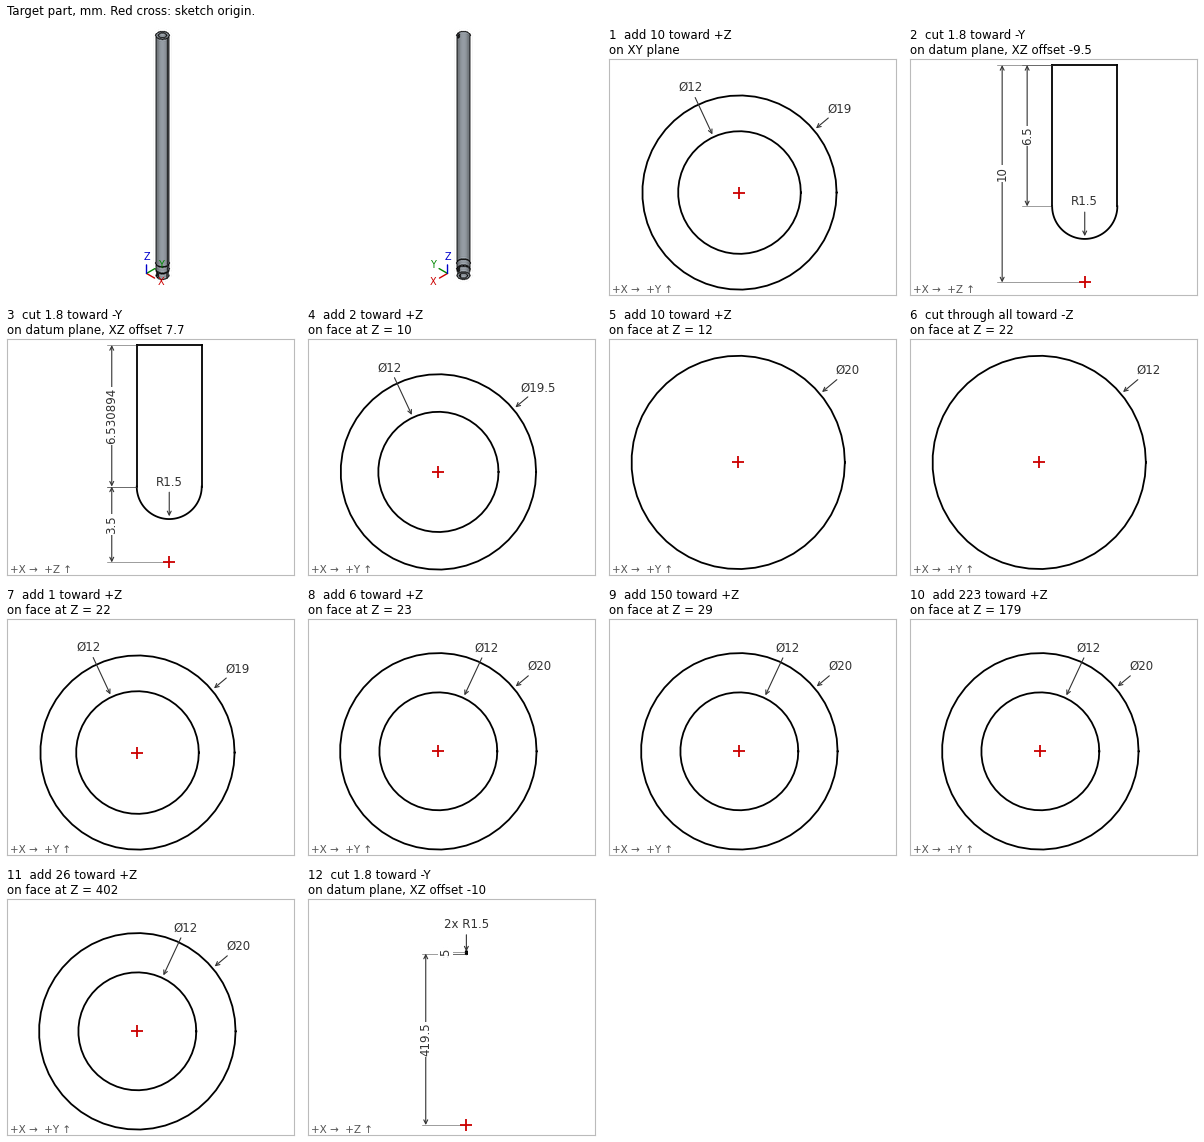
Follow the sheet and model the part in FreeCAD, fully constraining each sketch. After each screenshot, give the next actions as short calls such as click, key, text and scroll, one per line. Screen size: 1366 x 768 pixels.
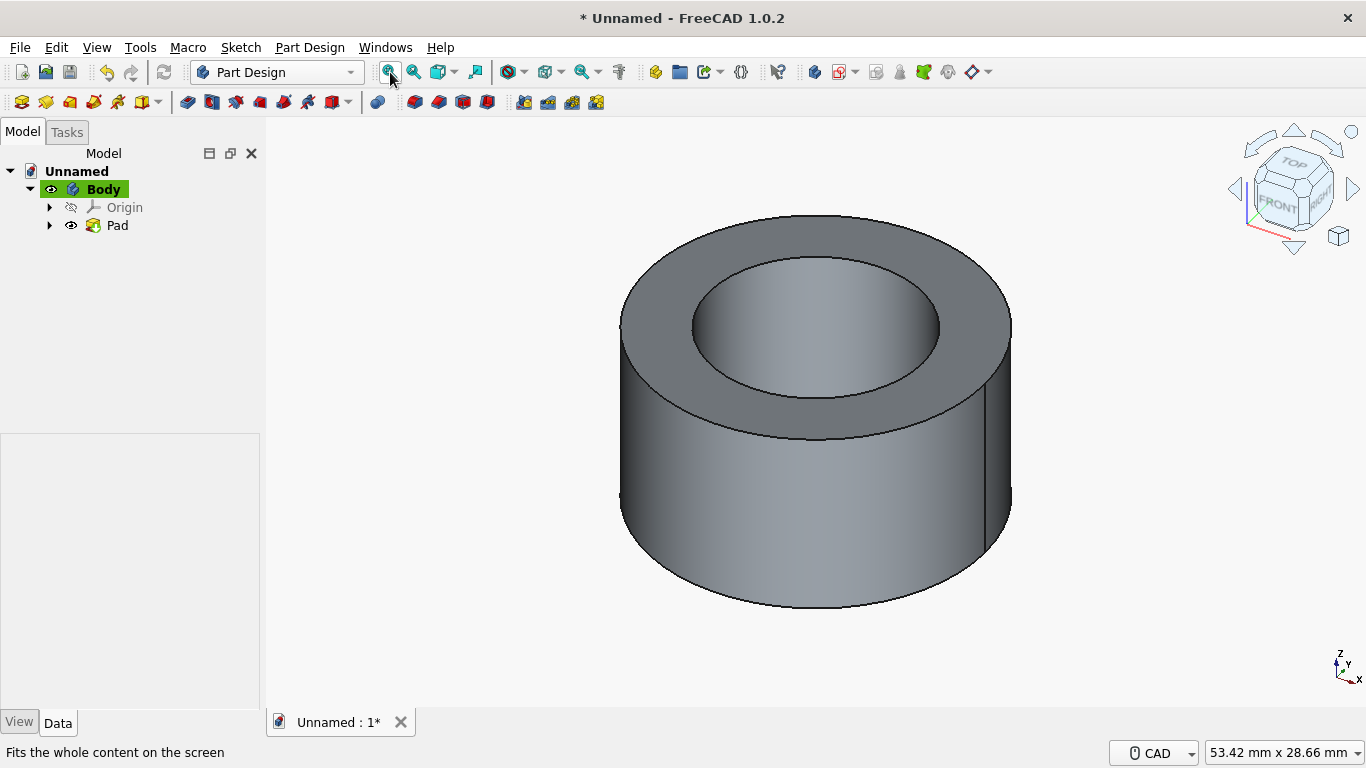
click(50, 207)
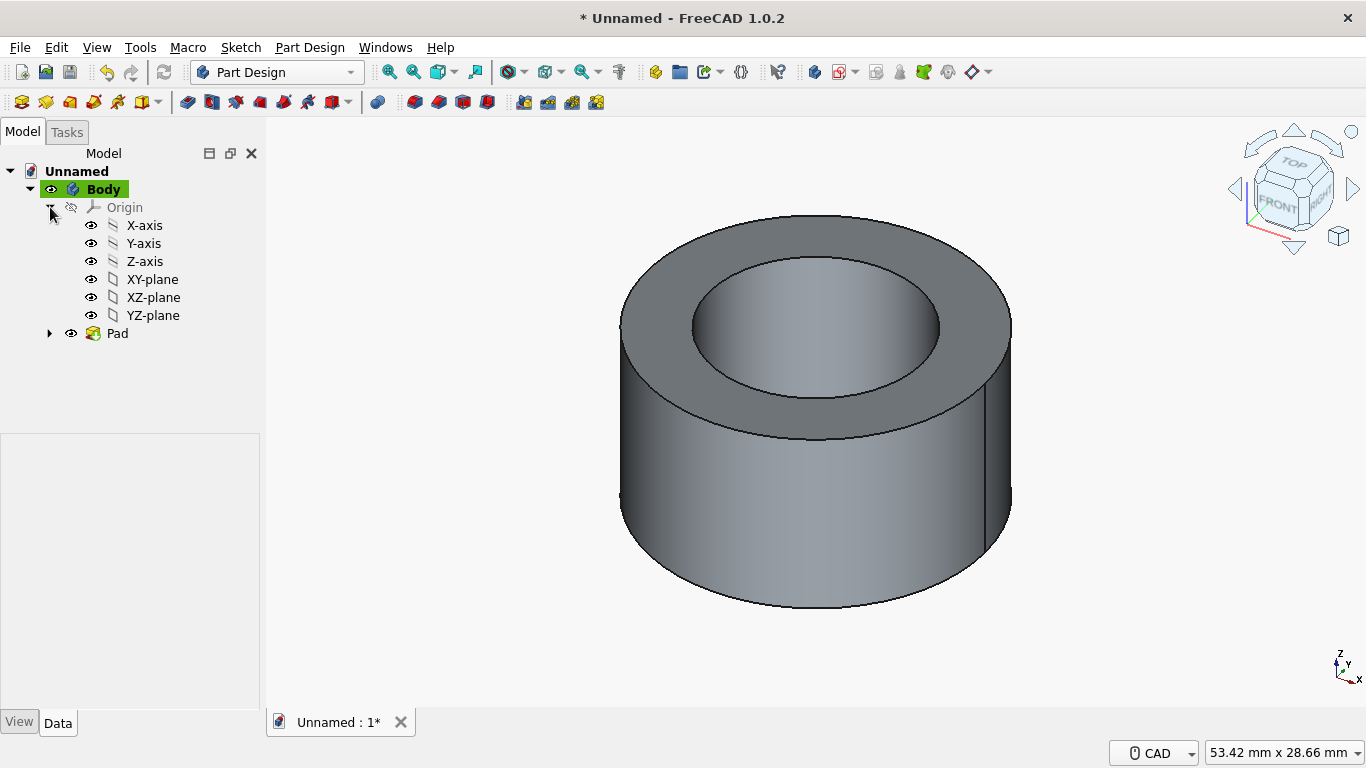
click(136, 297)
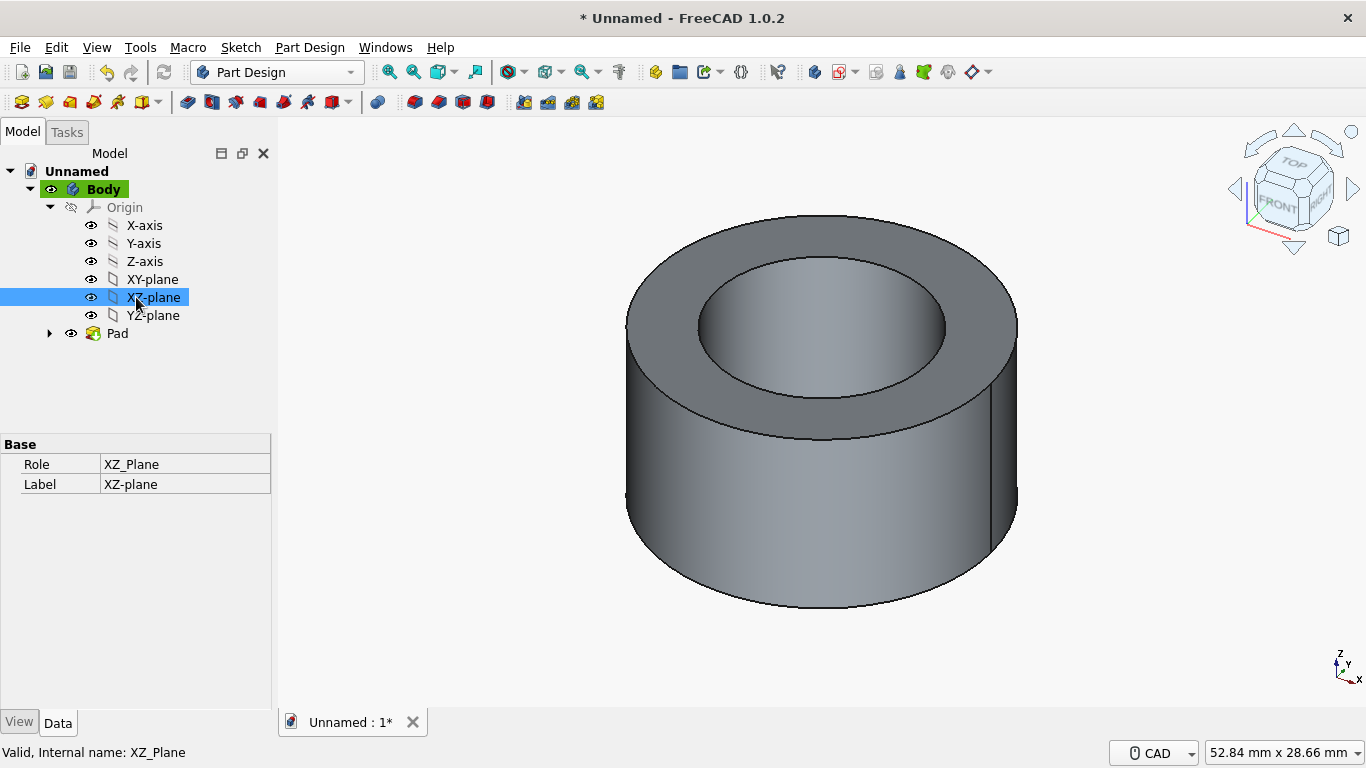
click(972, 72)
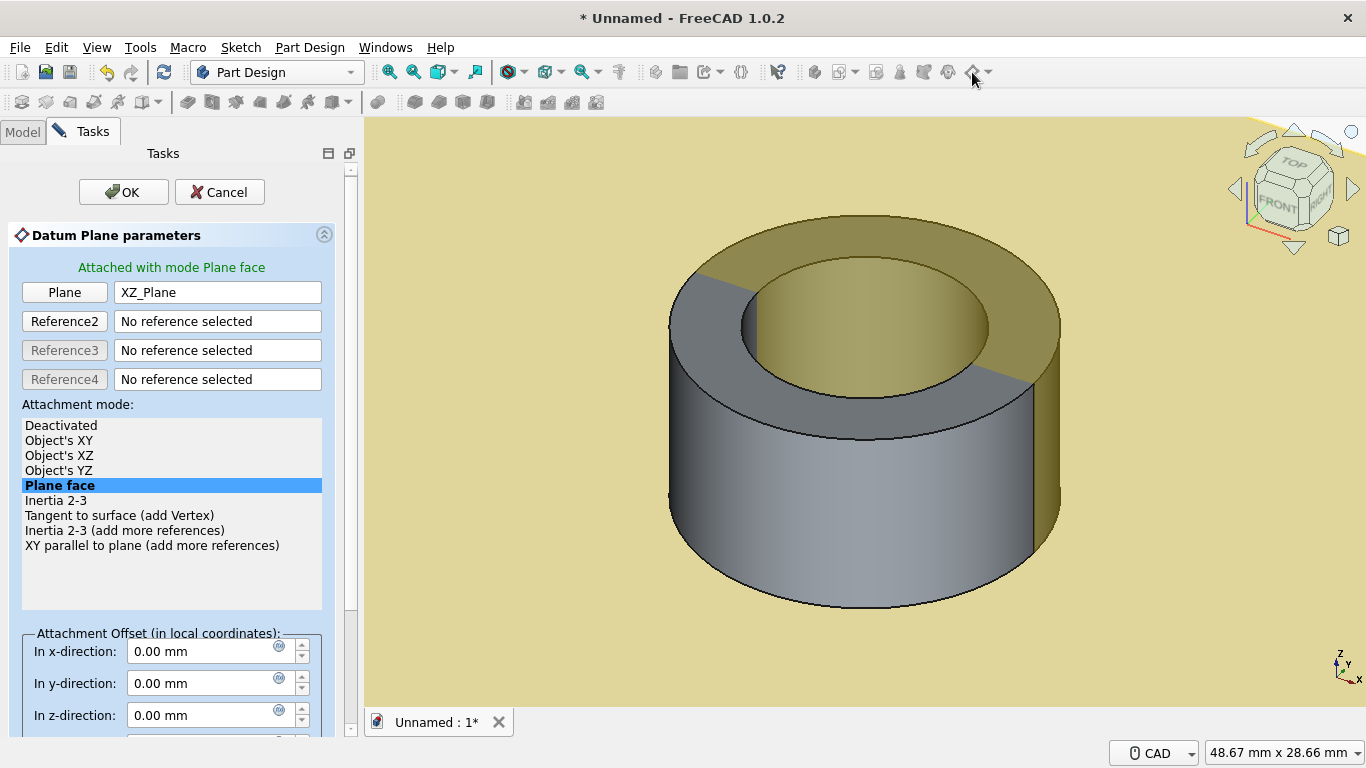
triple_click(210, 715)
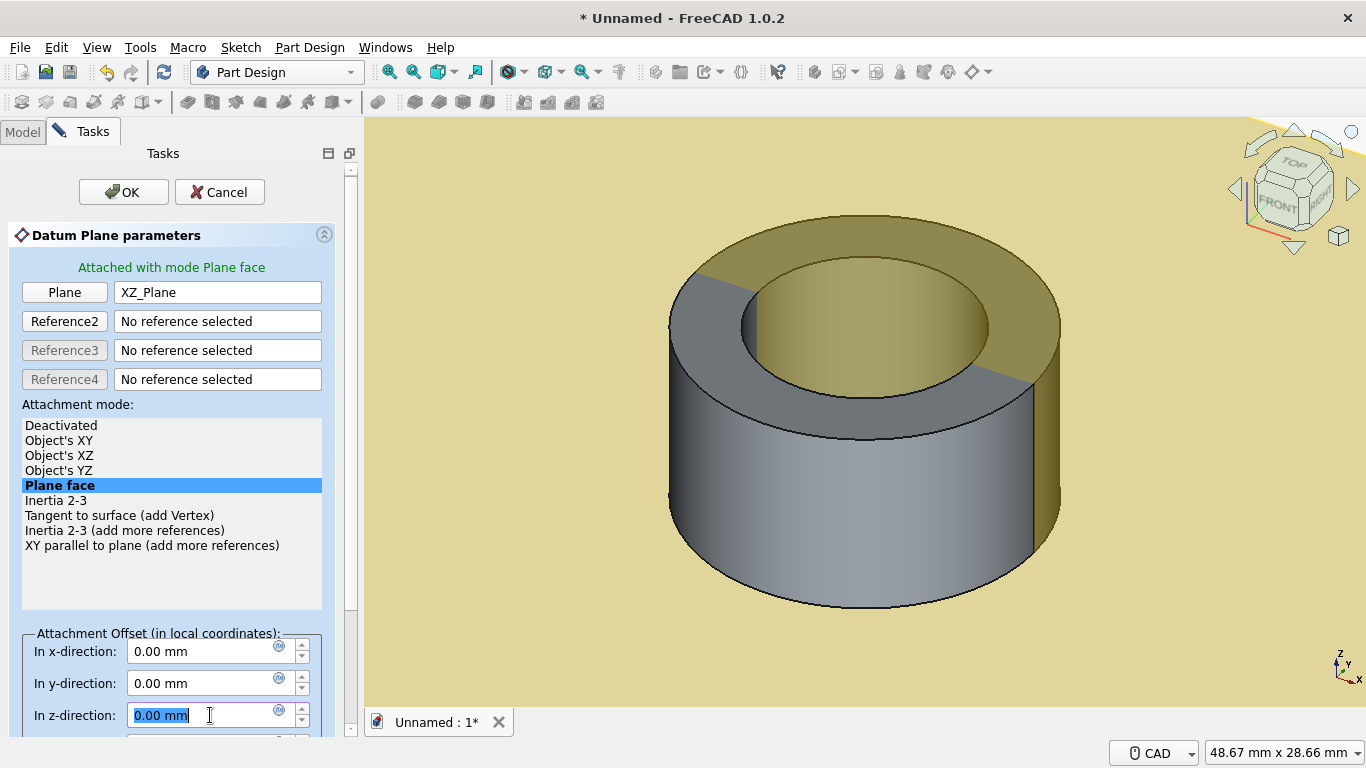
text(-9.5)
key(Tab)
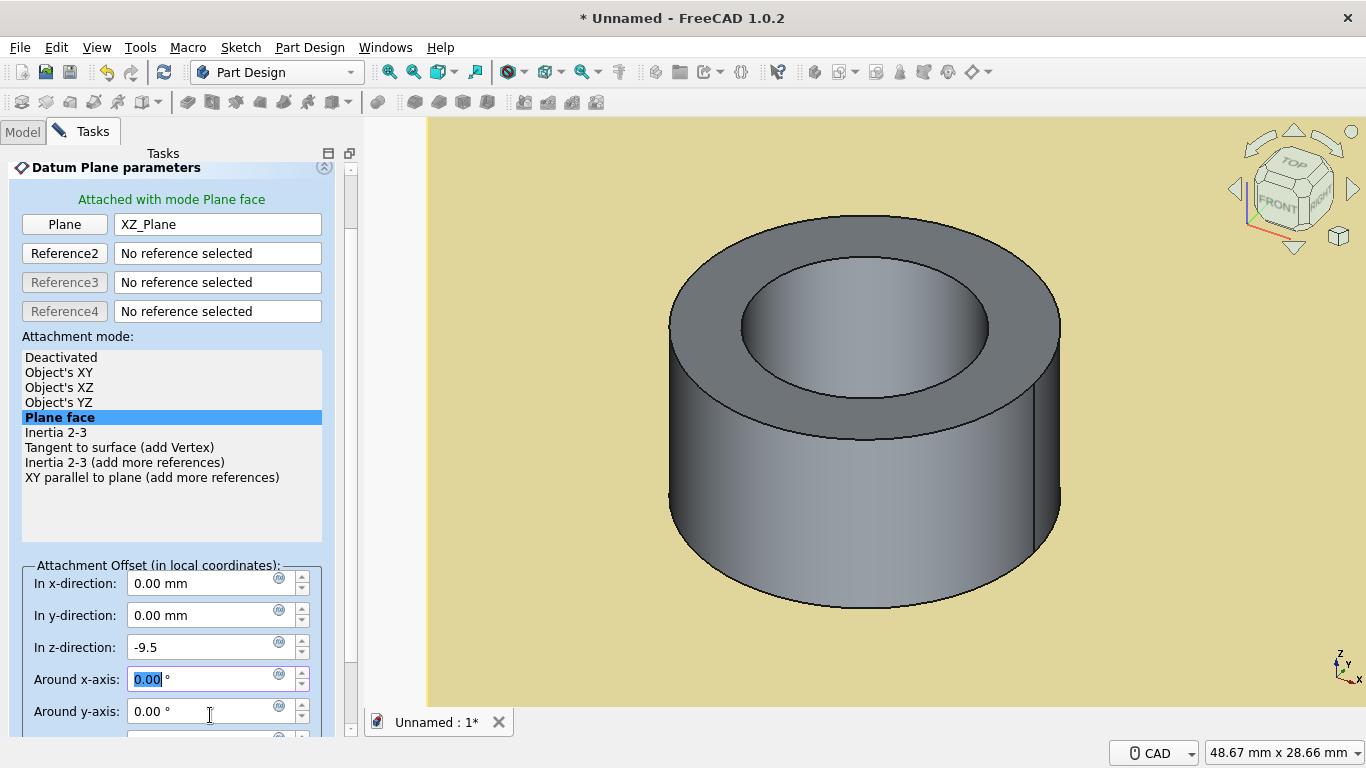
scroll(351, 450, up, 2)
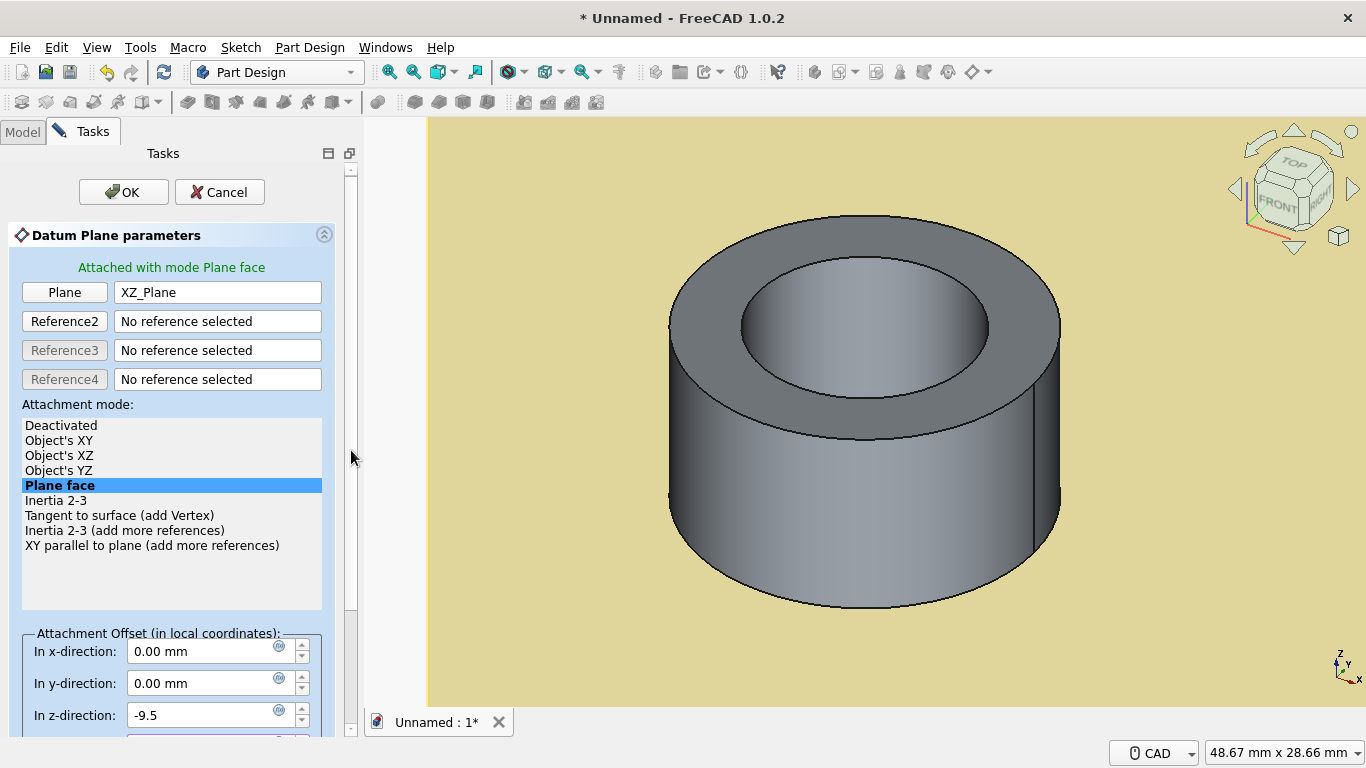
click(124, 192)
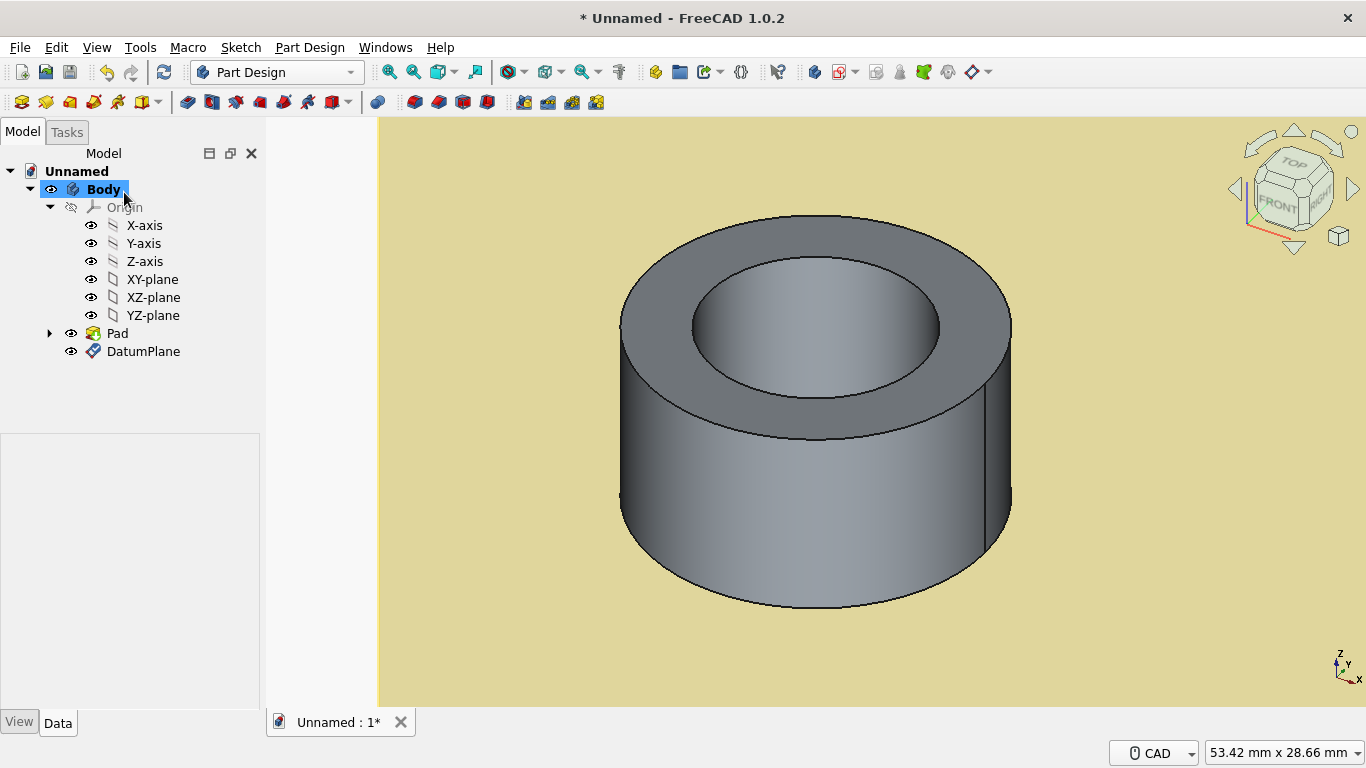
click(116, 351)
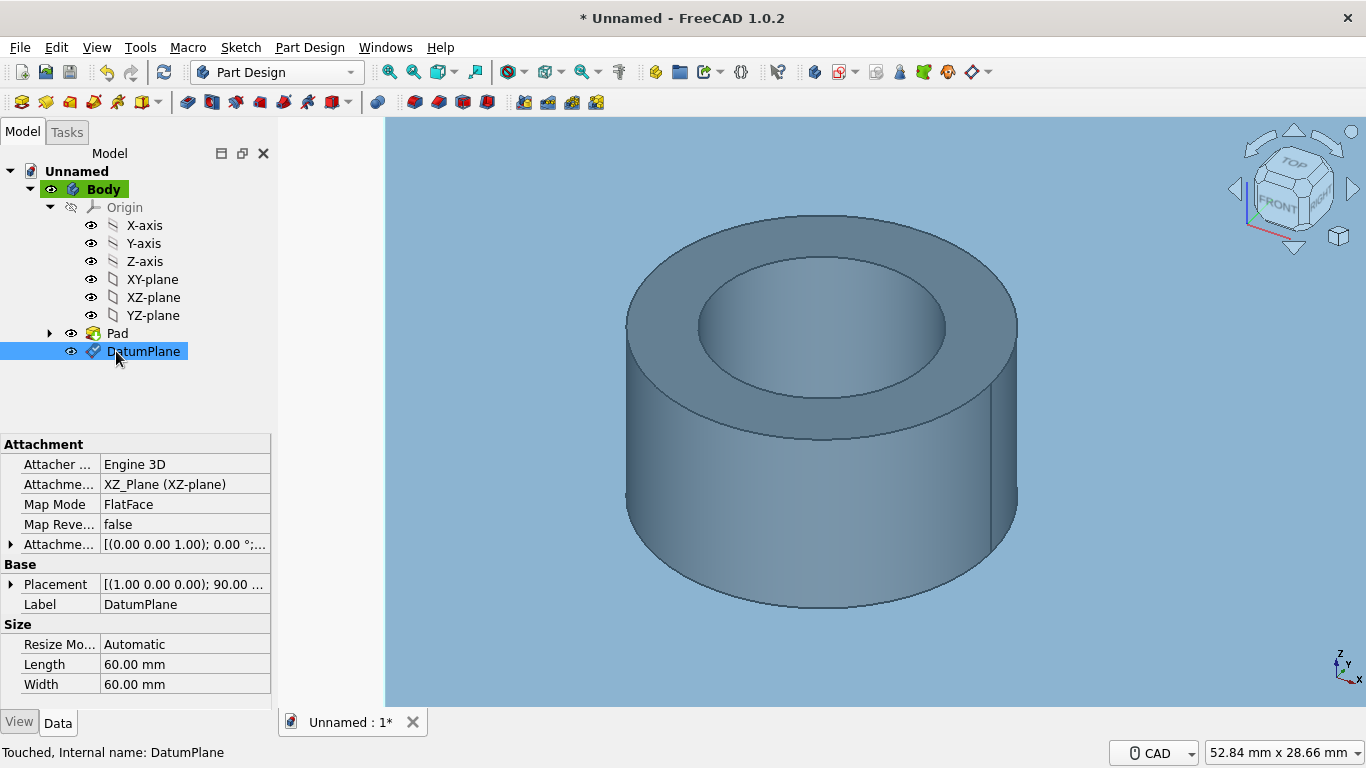
click(840, 72)